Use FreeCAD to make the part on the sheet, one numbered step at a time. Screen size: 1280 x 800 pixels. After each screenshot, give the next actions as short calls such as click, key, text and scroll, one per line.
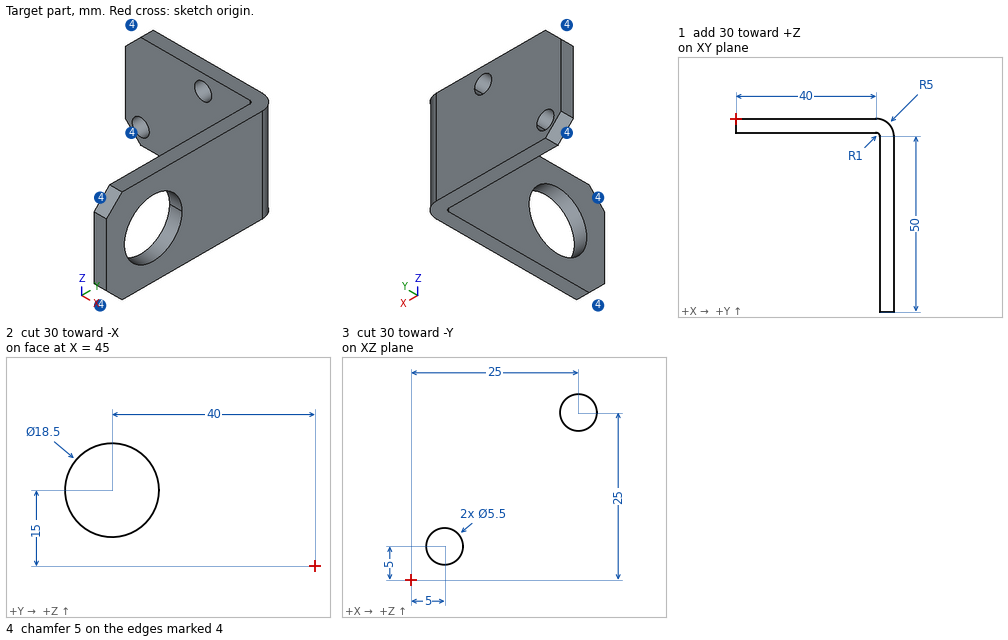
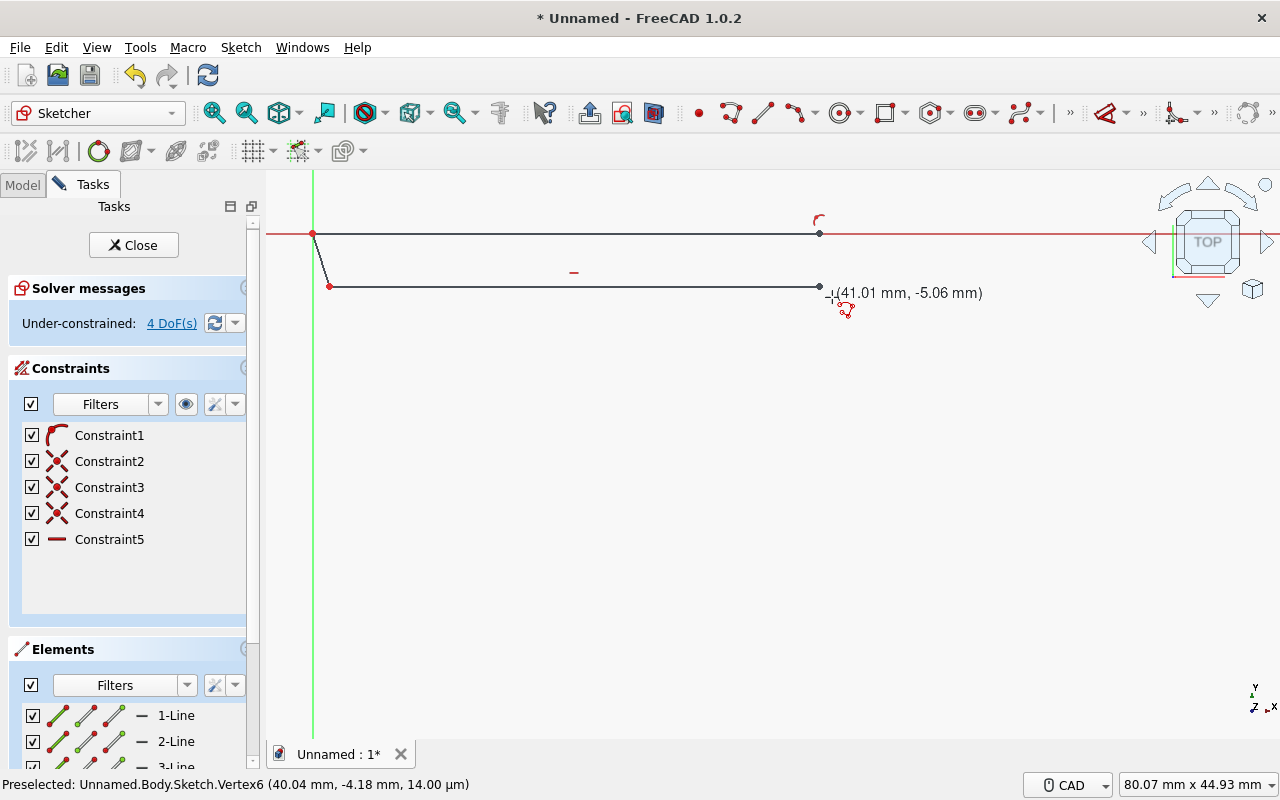
scroll(834, 299, down, 3)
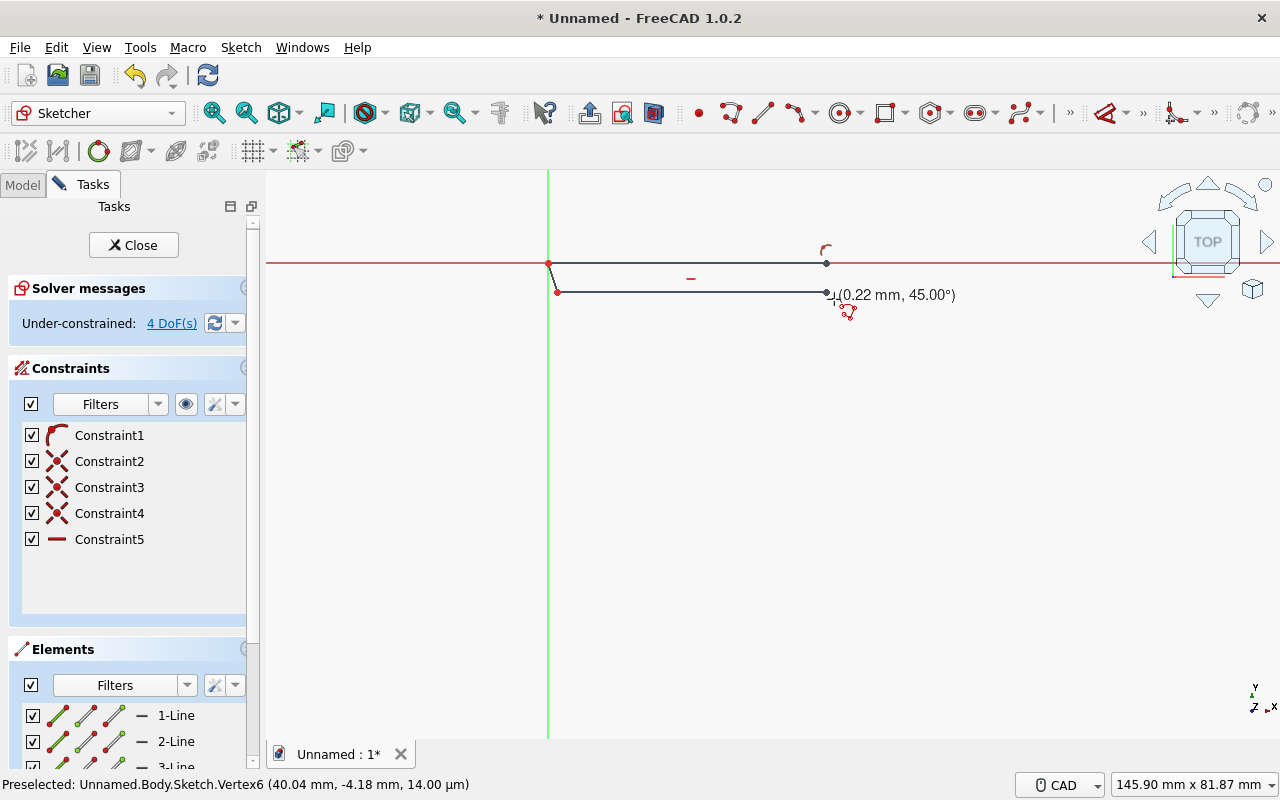
click(833, 646)
click(861, 646)
click(861, 298)
right_click(861, 298)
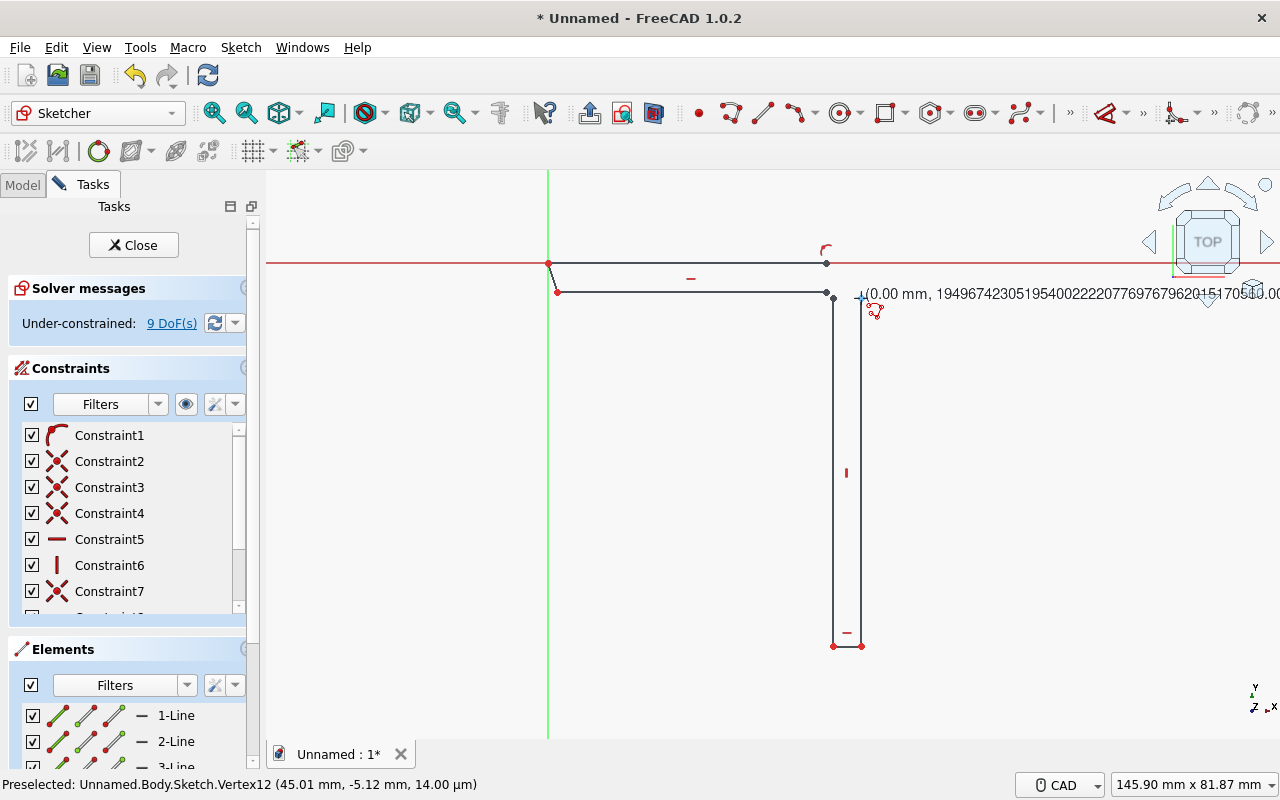
click(796, 114)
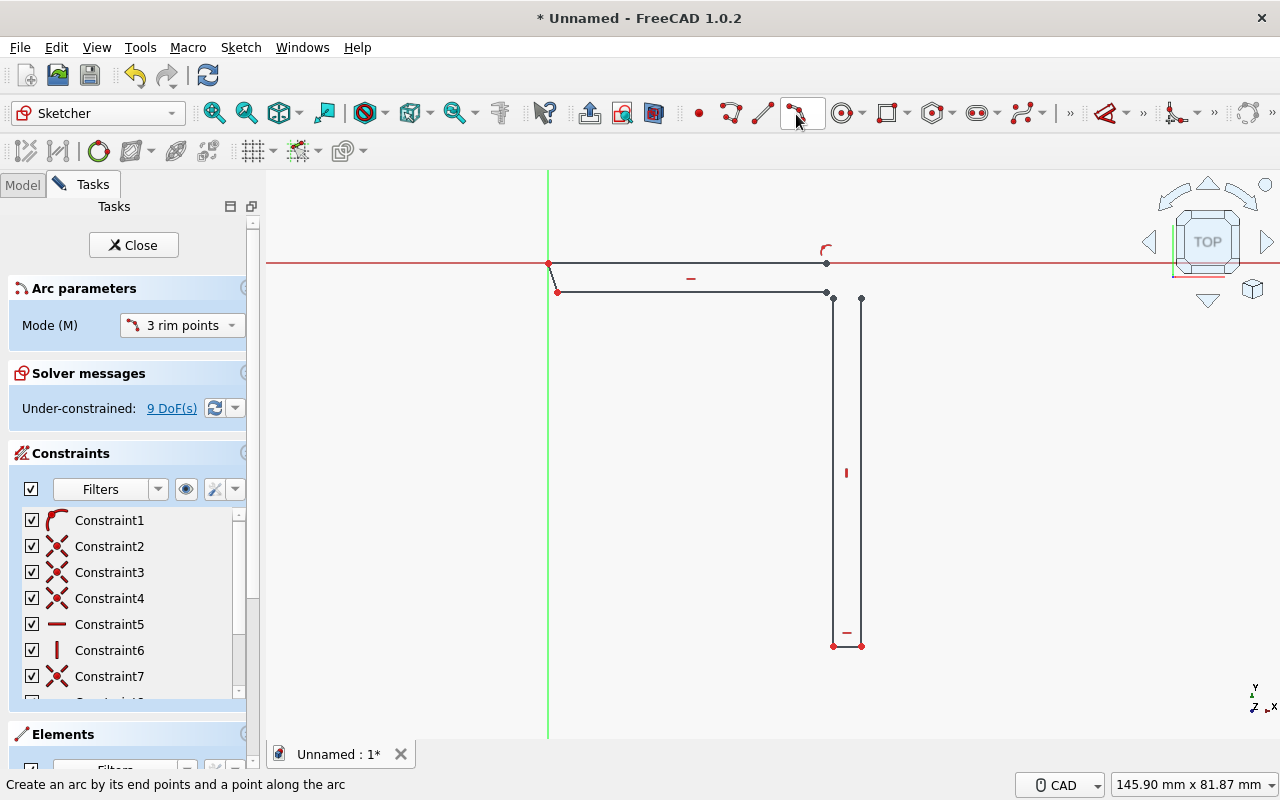
scroll(826, 291, up, 3)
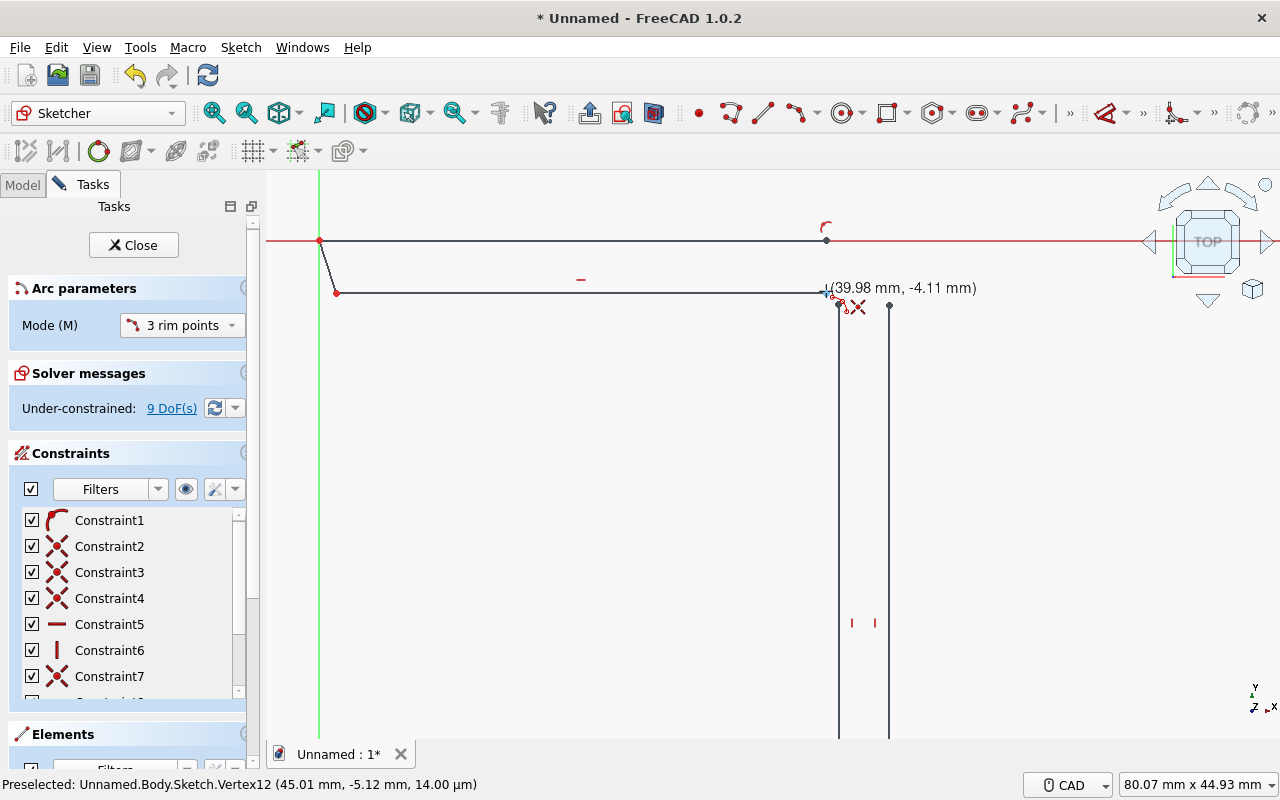
click(826, 293)
click(839, 305)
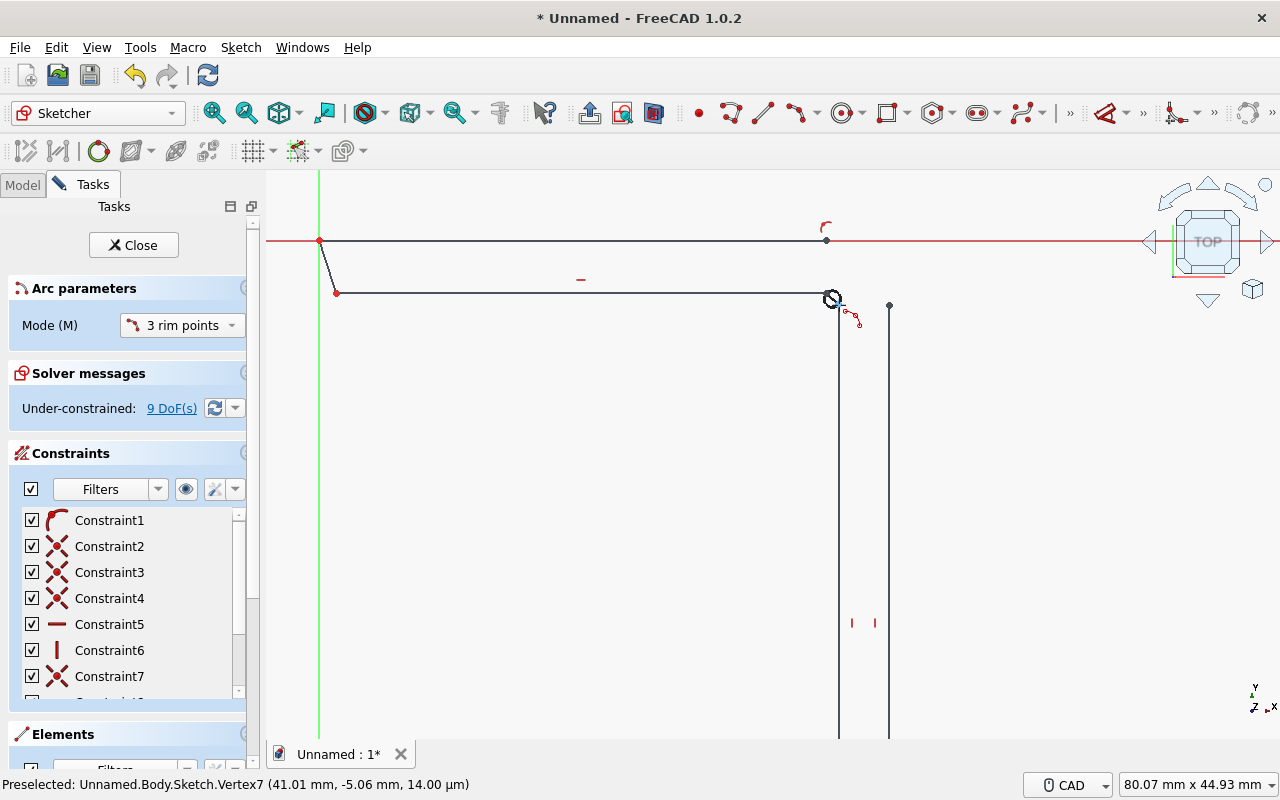
scroll(835, 295, up, 8)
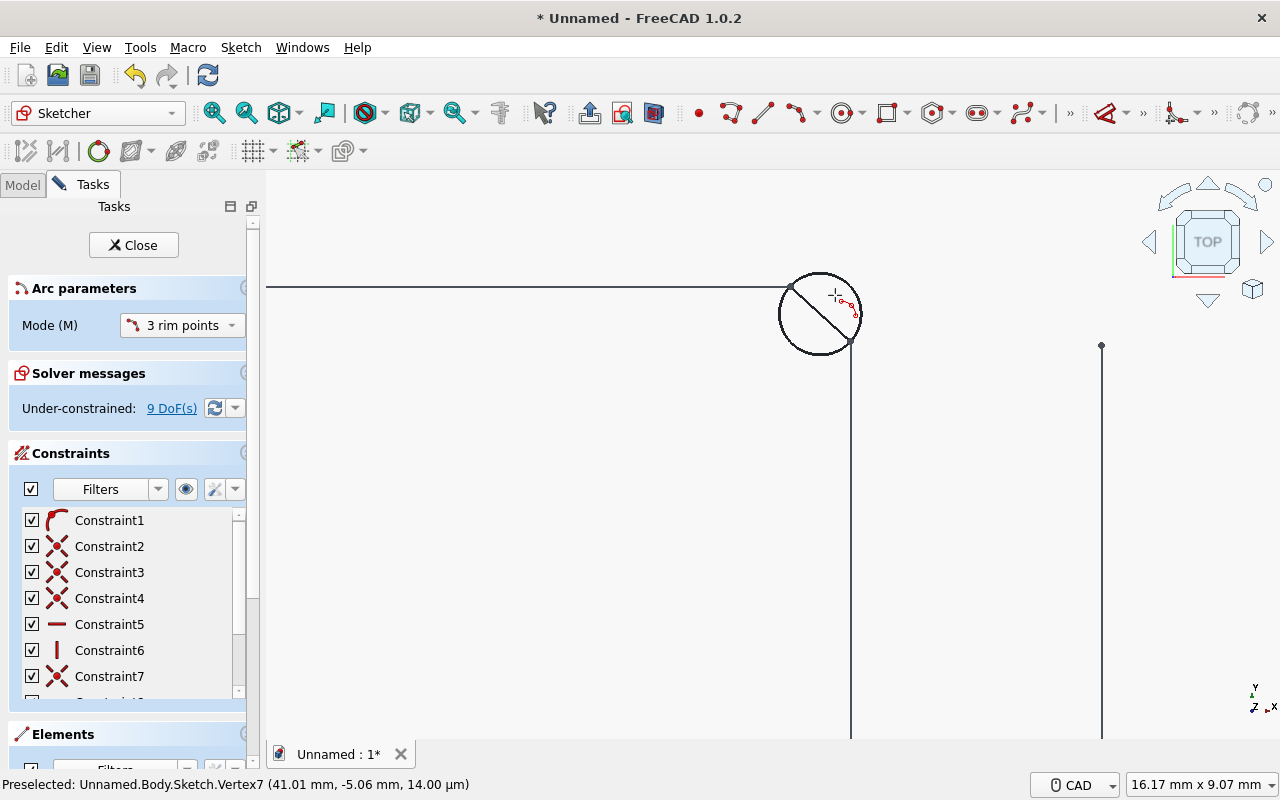
click(832, 294)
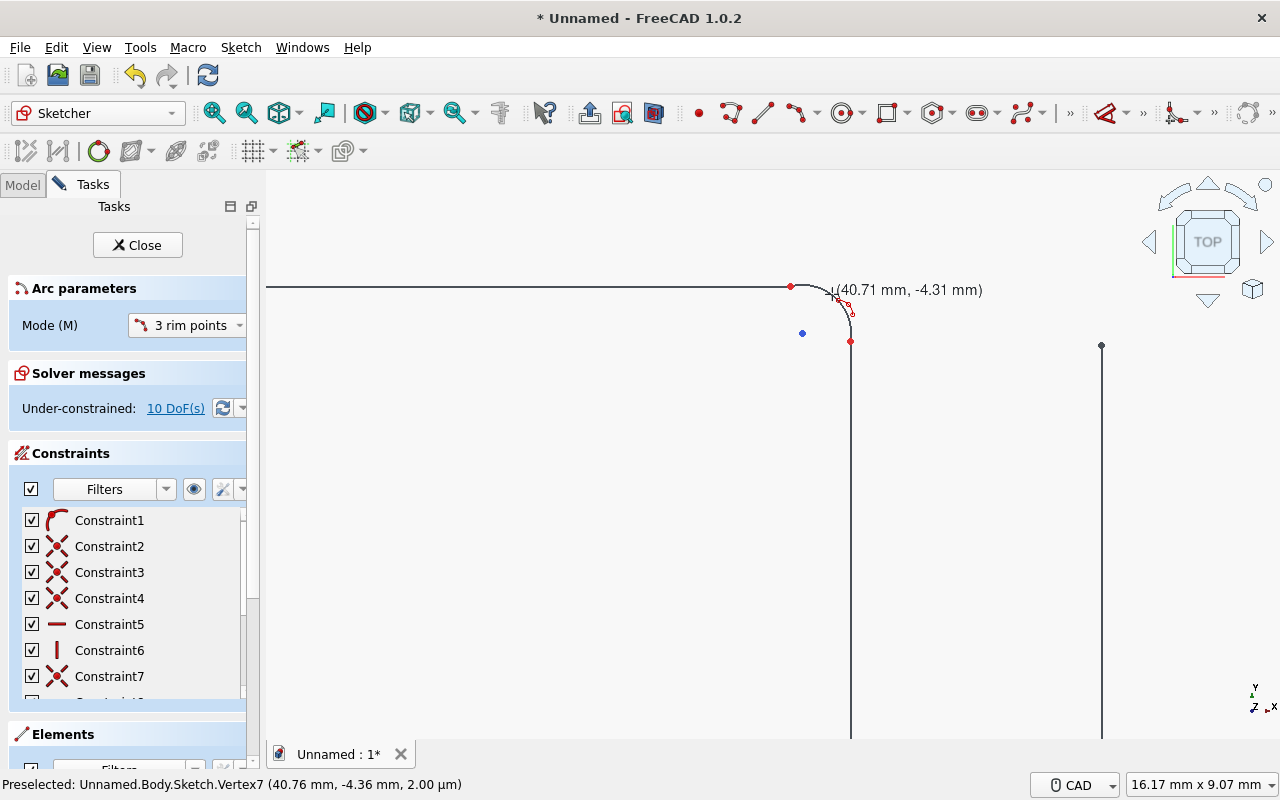
scroll(831, 293, down, 11)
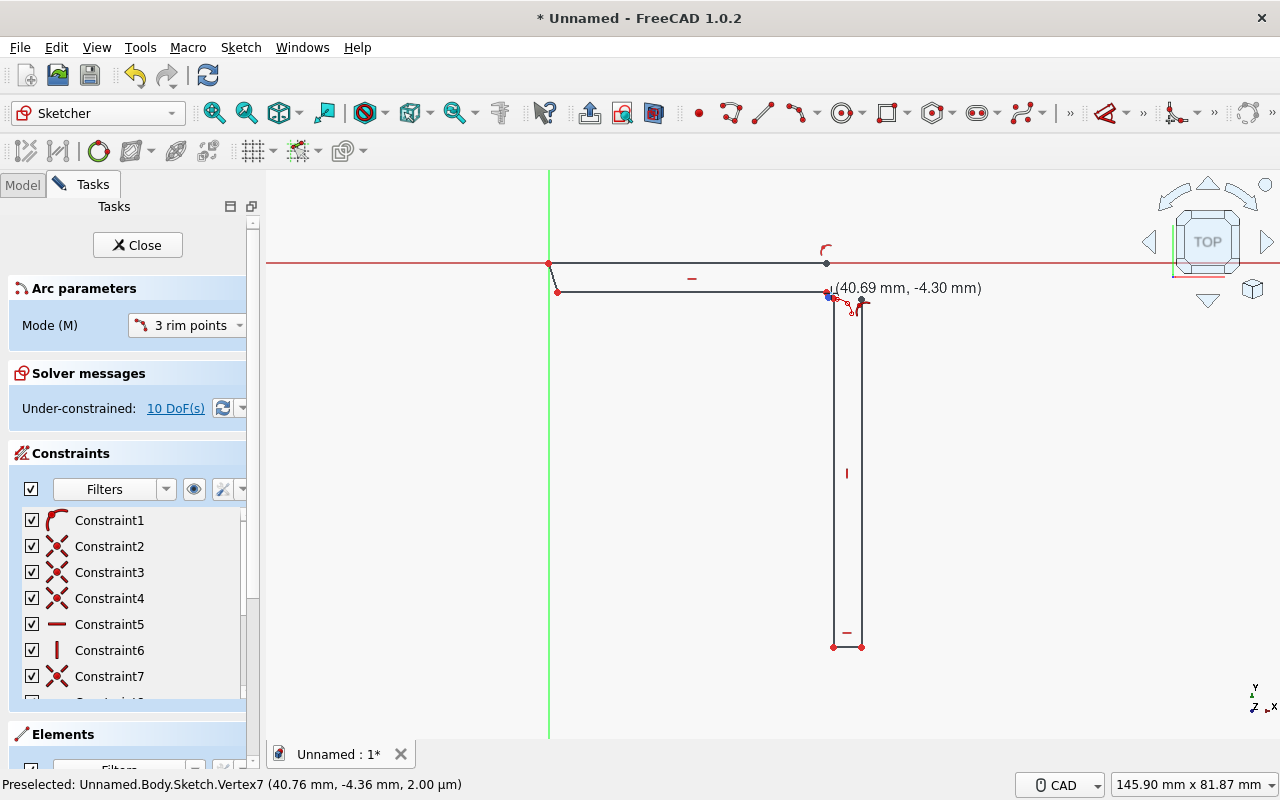
click(862, 299)
click(827, 263)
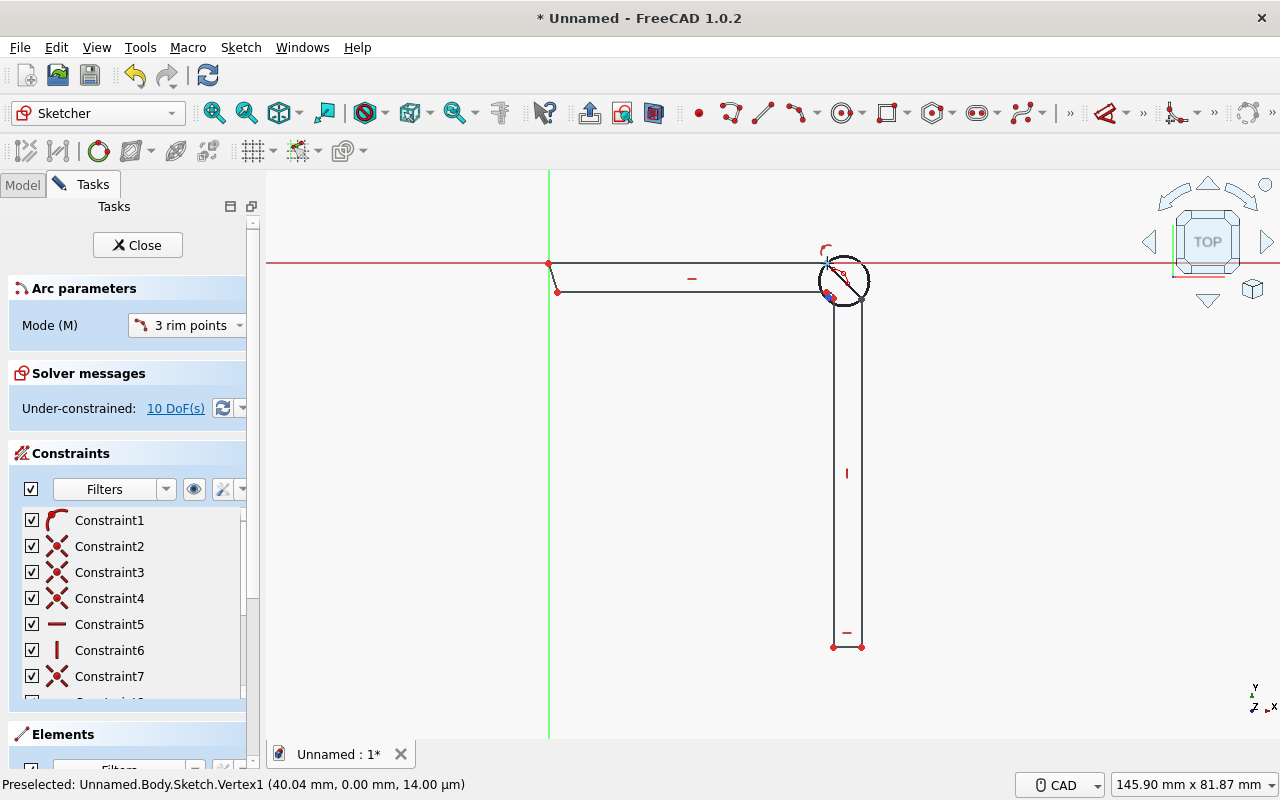
scroll(851, 274, up, 3)